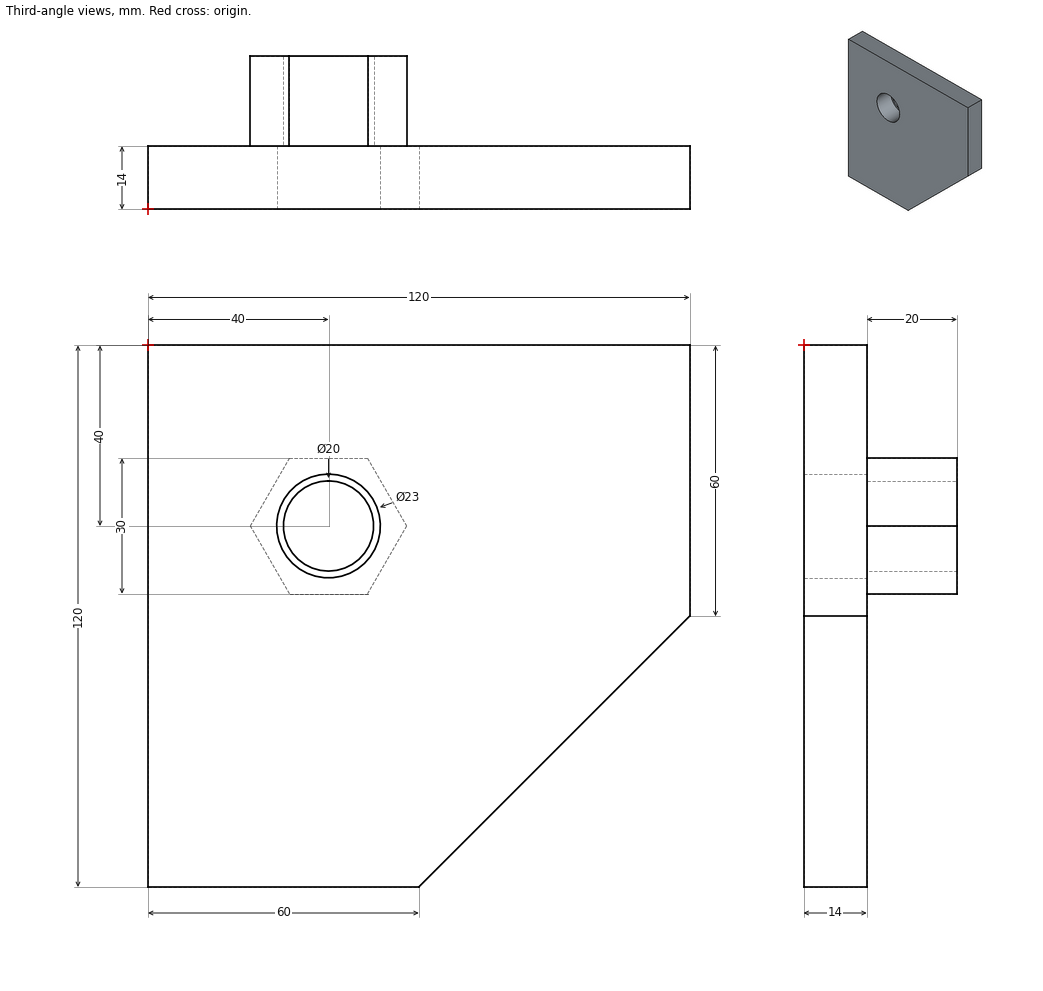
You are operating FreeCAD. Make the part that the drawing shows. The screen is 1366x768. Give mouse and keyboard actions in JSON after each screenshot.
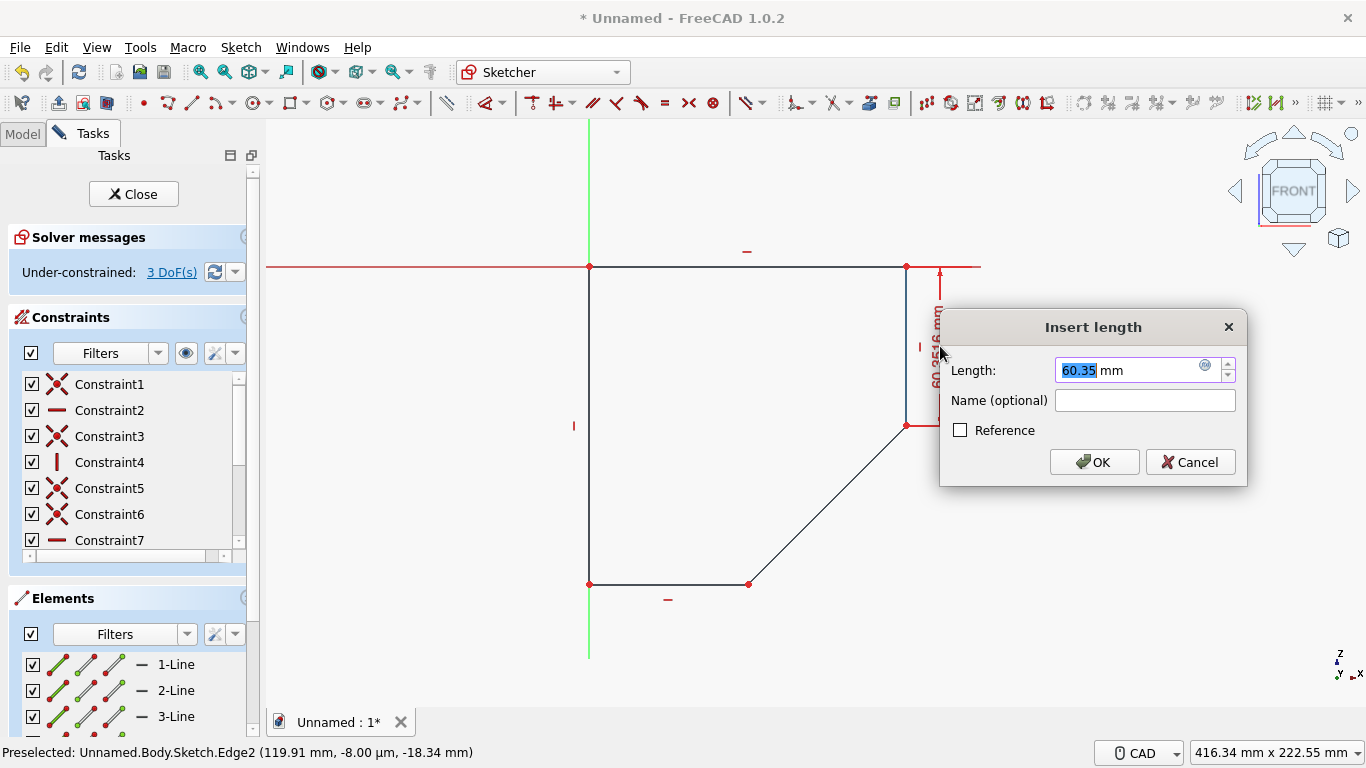
{"action": "type", "text": "60"}
{"action": "key", "text": "Return"}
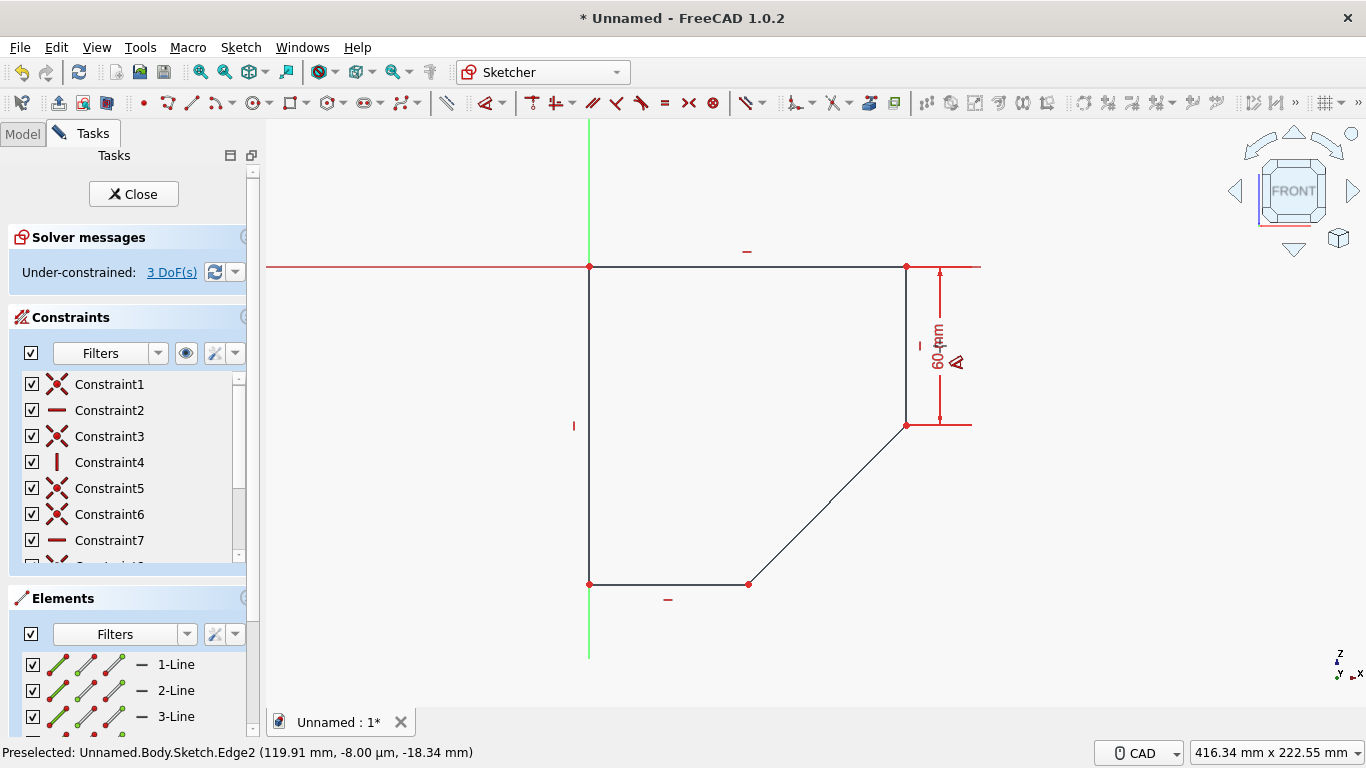
{"action": "left_click", "coordinate": [700, 585]}
{"action": "left_click", "coordinate": [669, 619]}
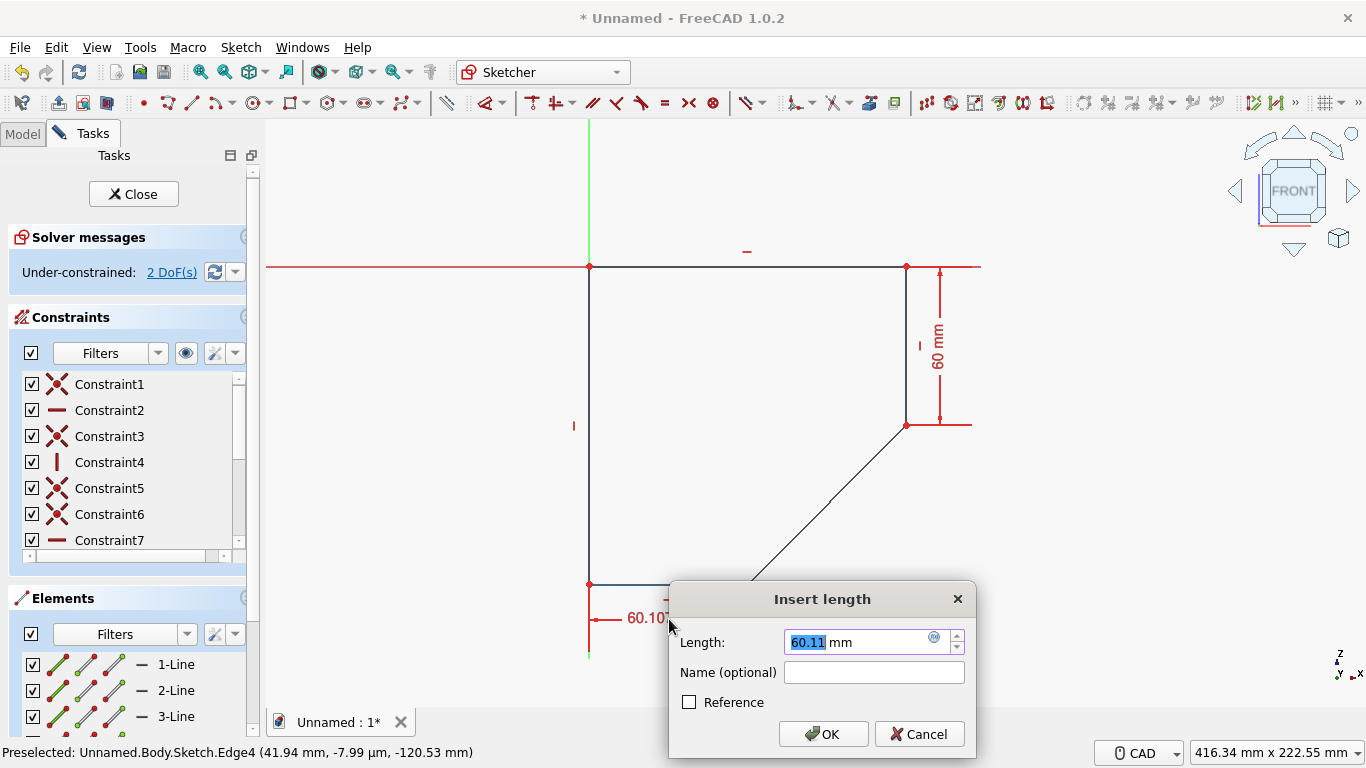
{"action": "type", "text": "60"}
{"action": "key", "text": "Return"}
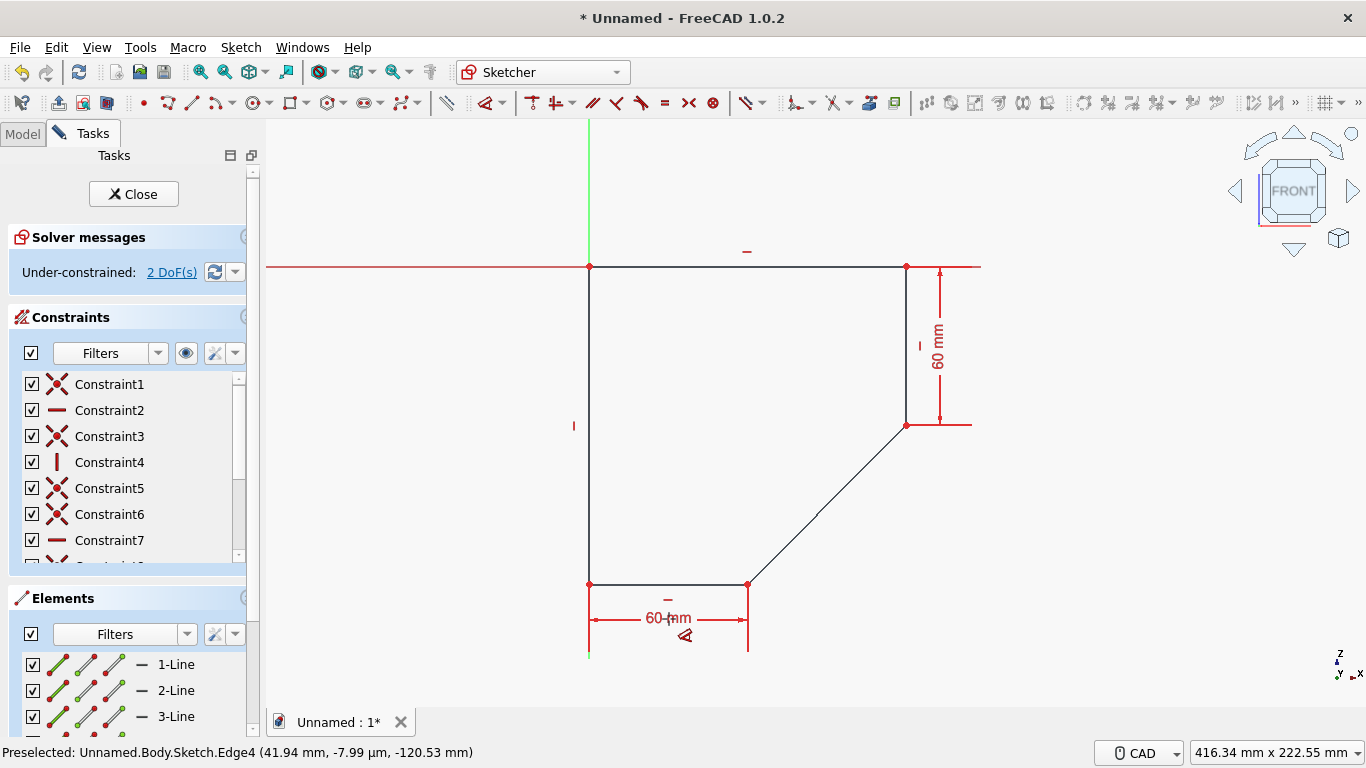
{"action": "left_click", "coordinate": [684, 267]}
{"action": "left_click", "coordinate": [748, 233]}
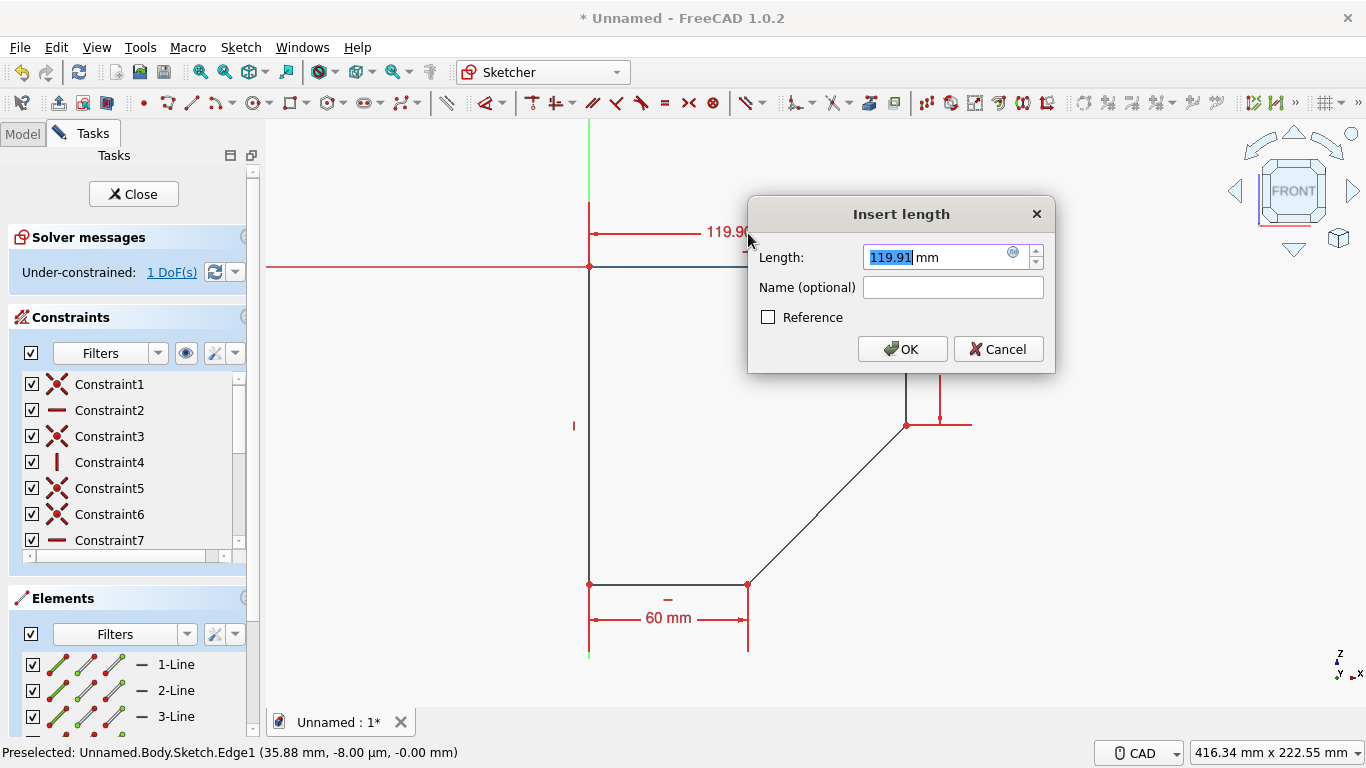
{"action": "type", "text": "120"}
{"action": "key", "text": "Return"}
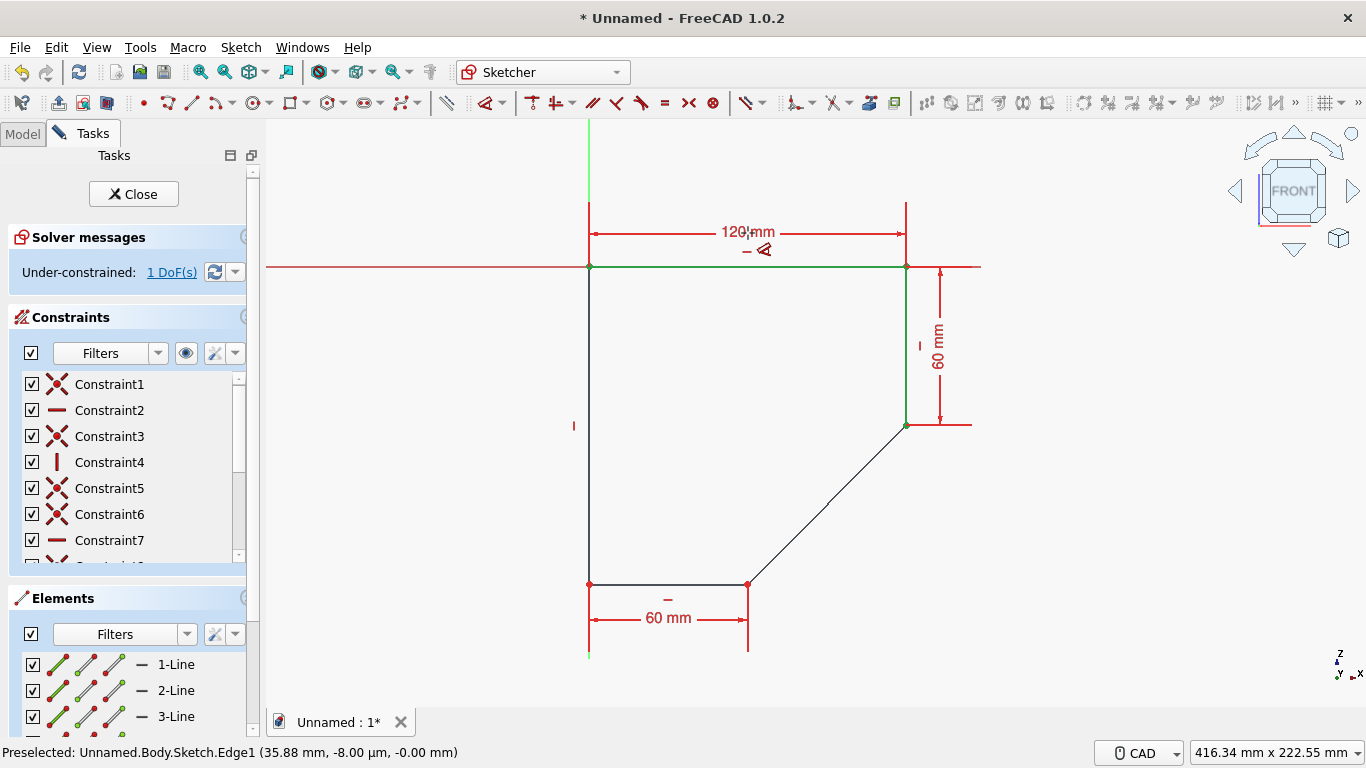
{"action": "left_click", "coordinate": [589, 489]}
{"action": "left_click", "coordinate": [555, 426]}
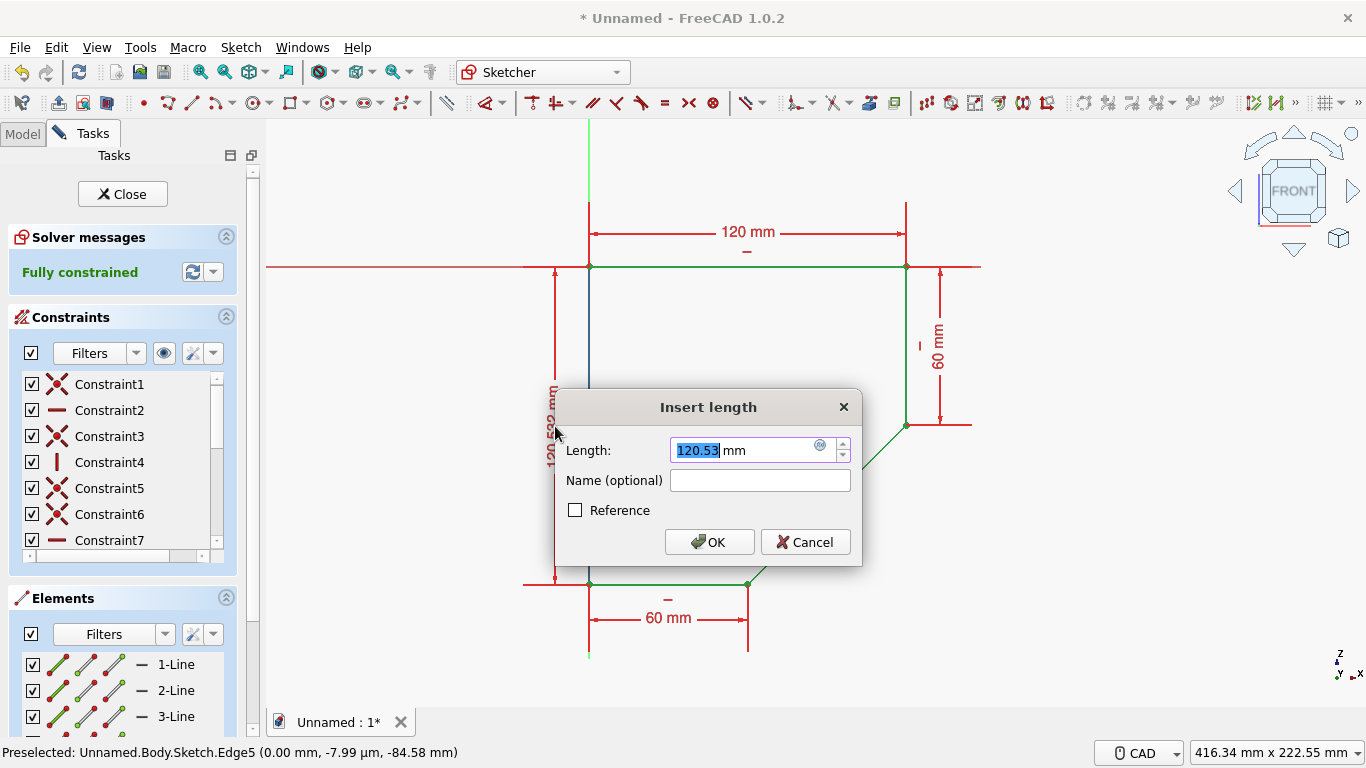
{"action": "type", "text": "120"}
{"action": "key", "text": "Return"}
{"action": "key", "text": "Escape"}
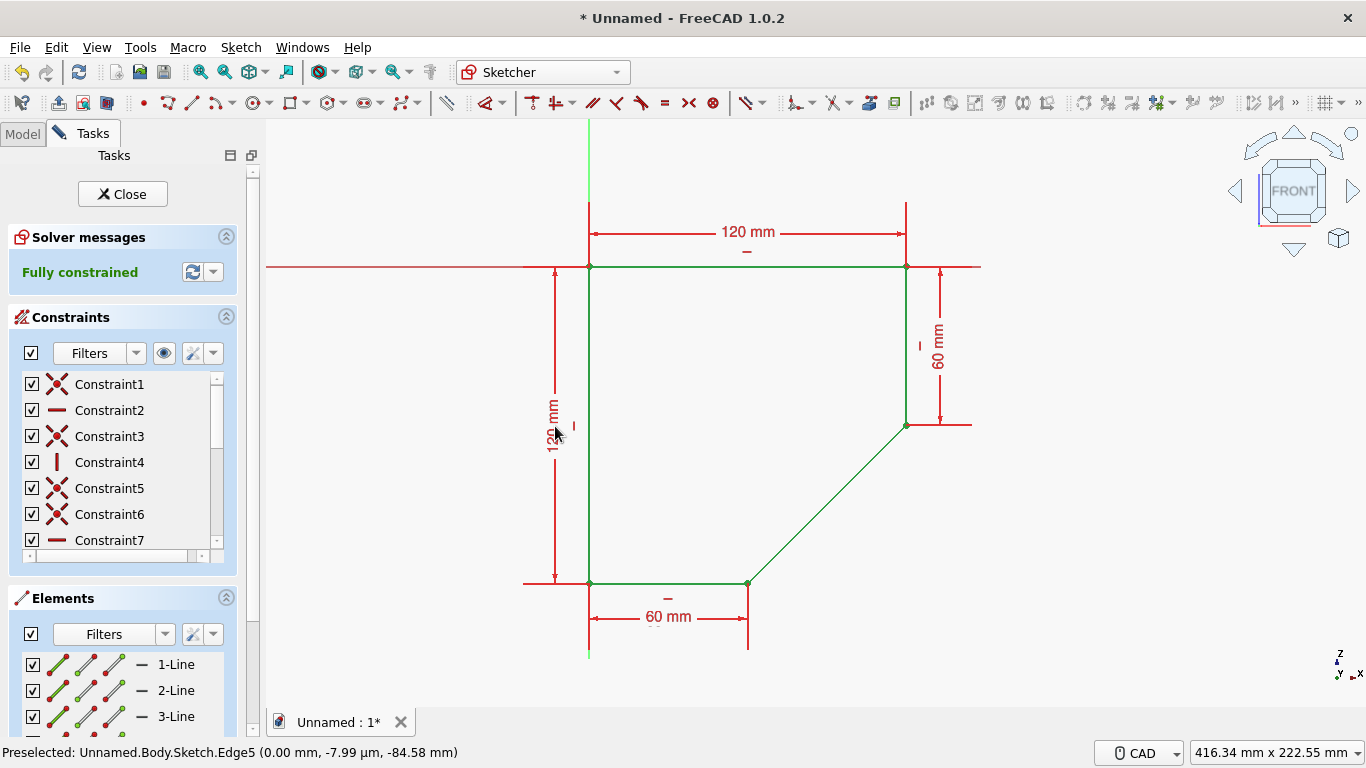
{"action": "left_click", "coordinate": [123, 194]}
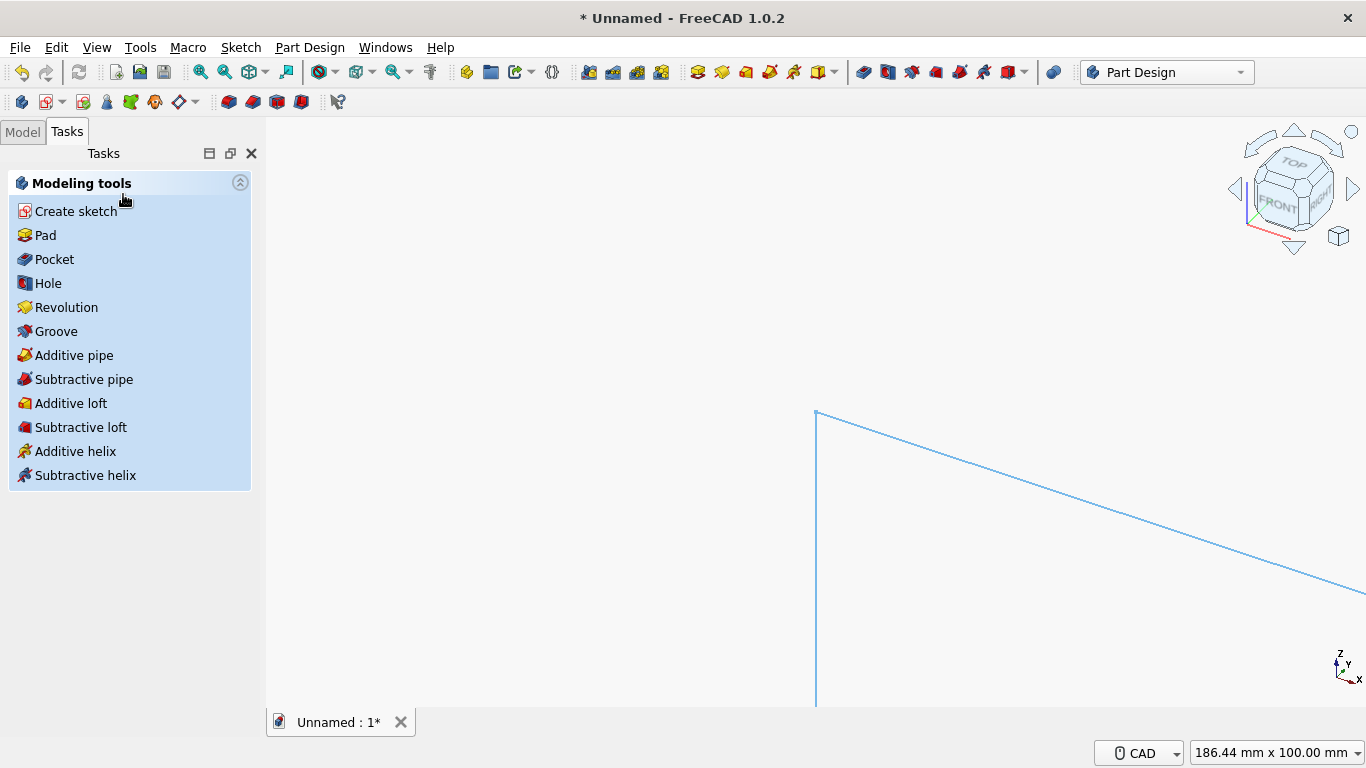
{"action": "left_click", "coordinate": [698, 72]}